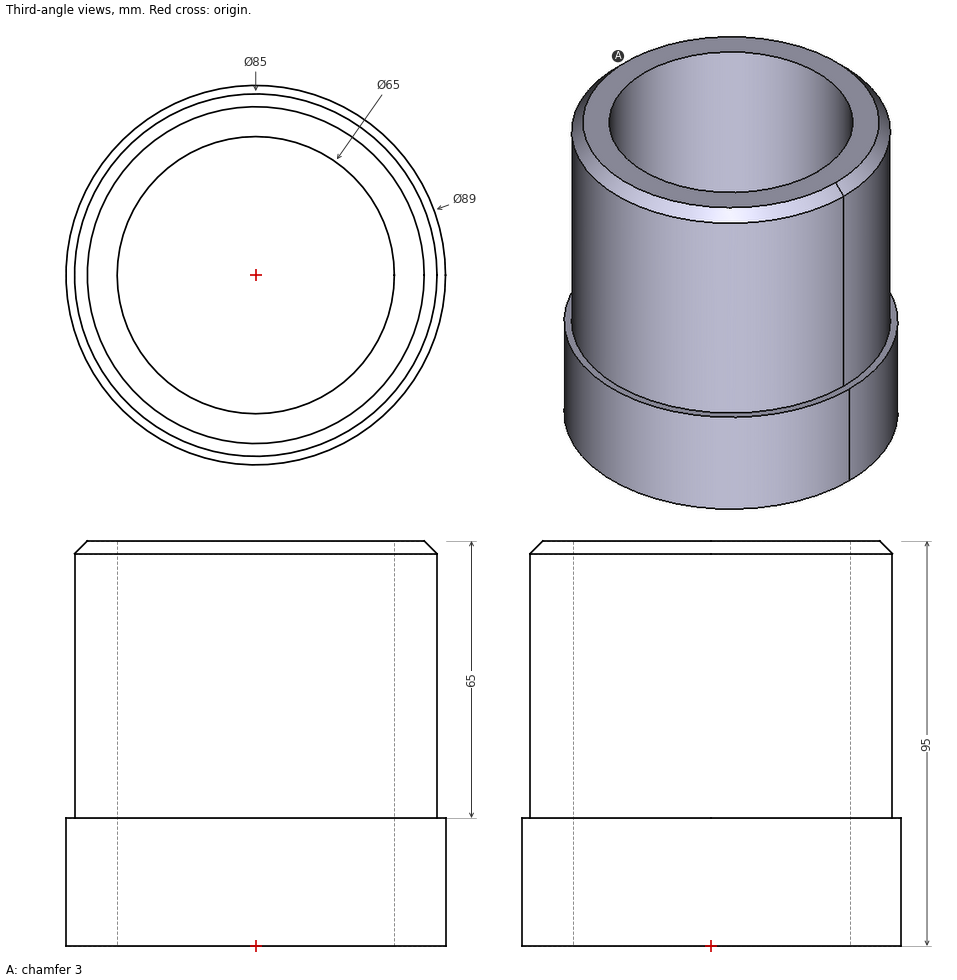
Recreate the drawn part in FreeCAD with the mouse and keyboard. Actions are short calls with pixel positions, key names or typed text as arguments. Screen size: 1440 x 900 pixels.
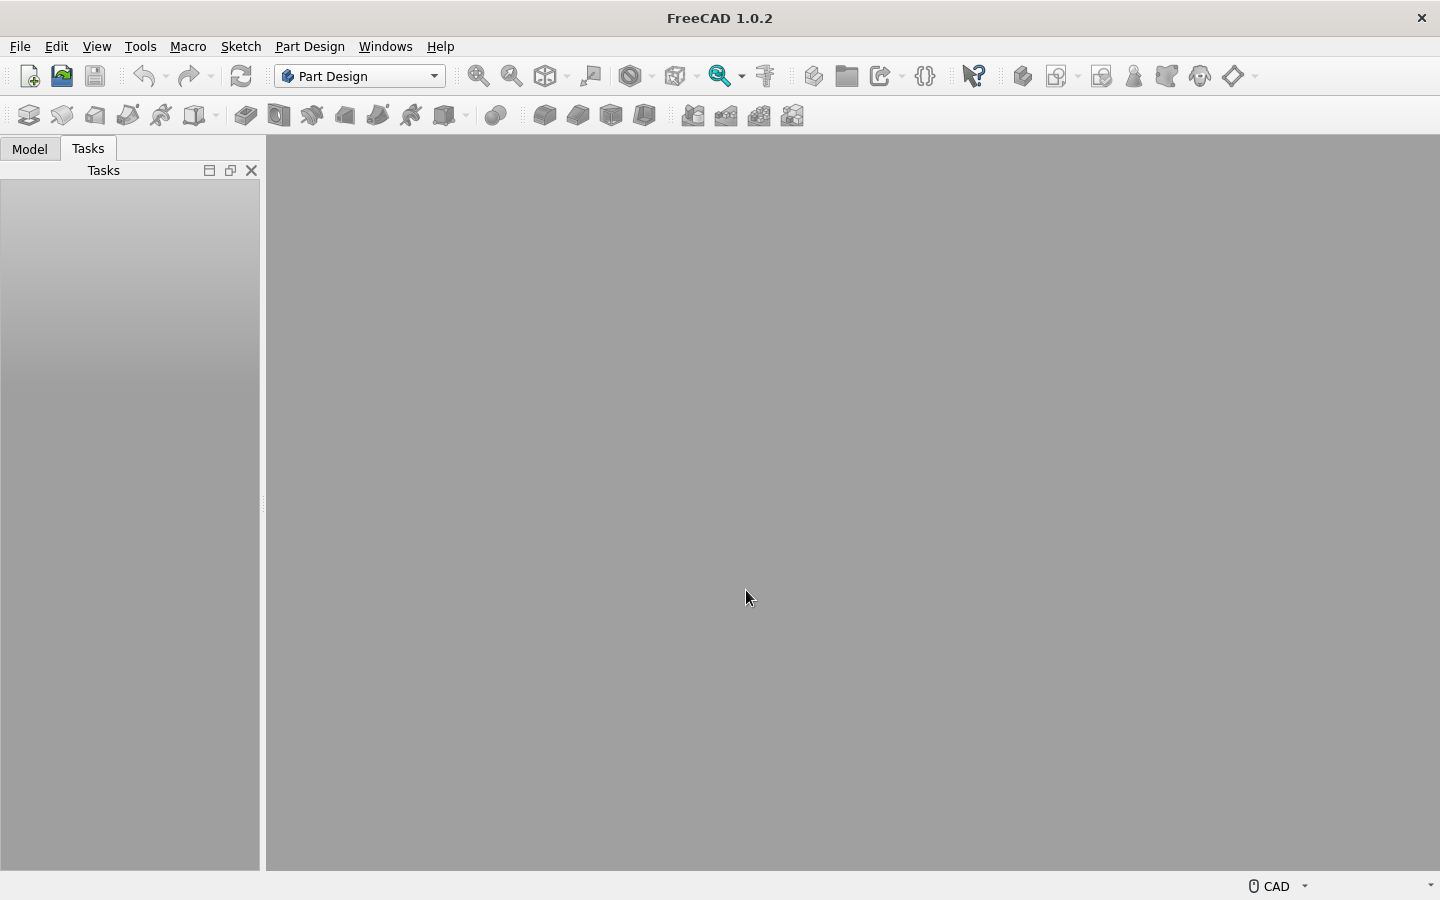
click(29, 76)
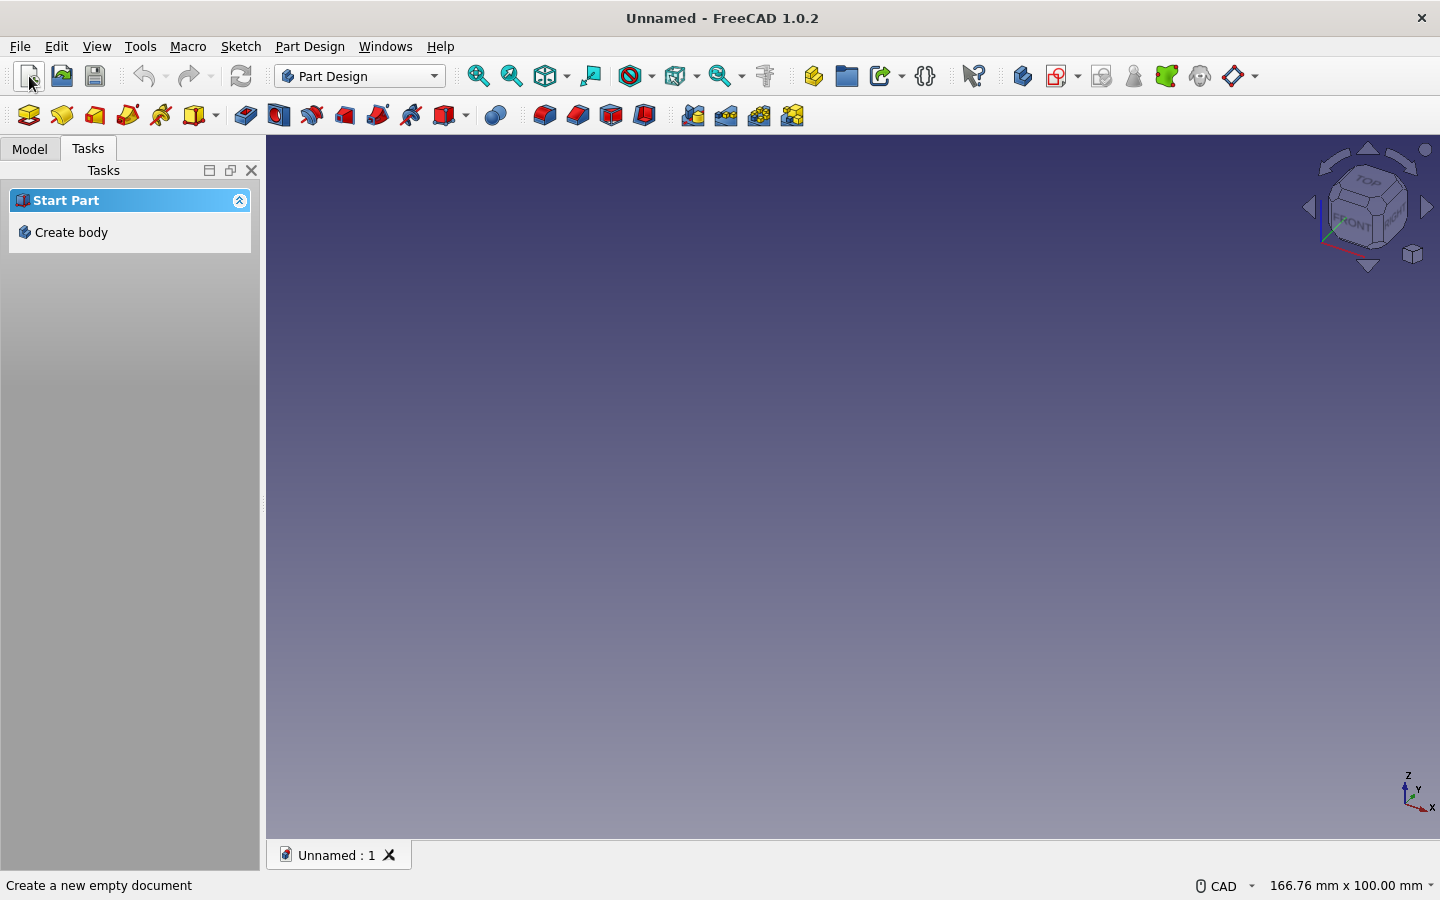
click(1056, 76)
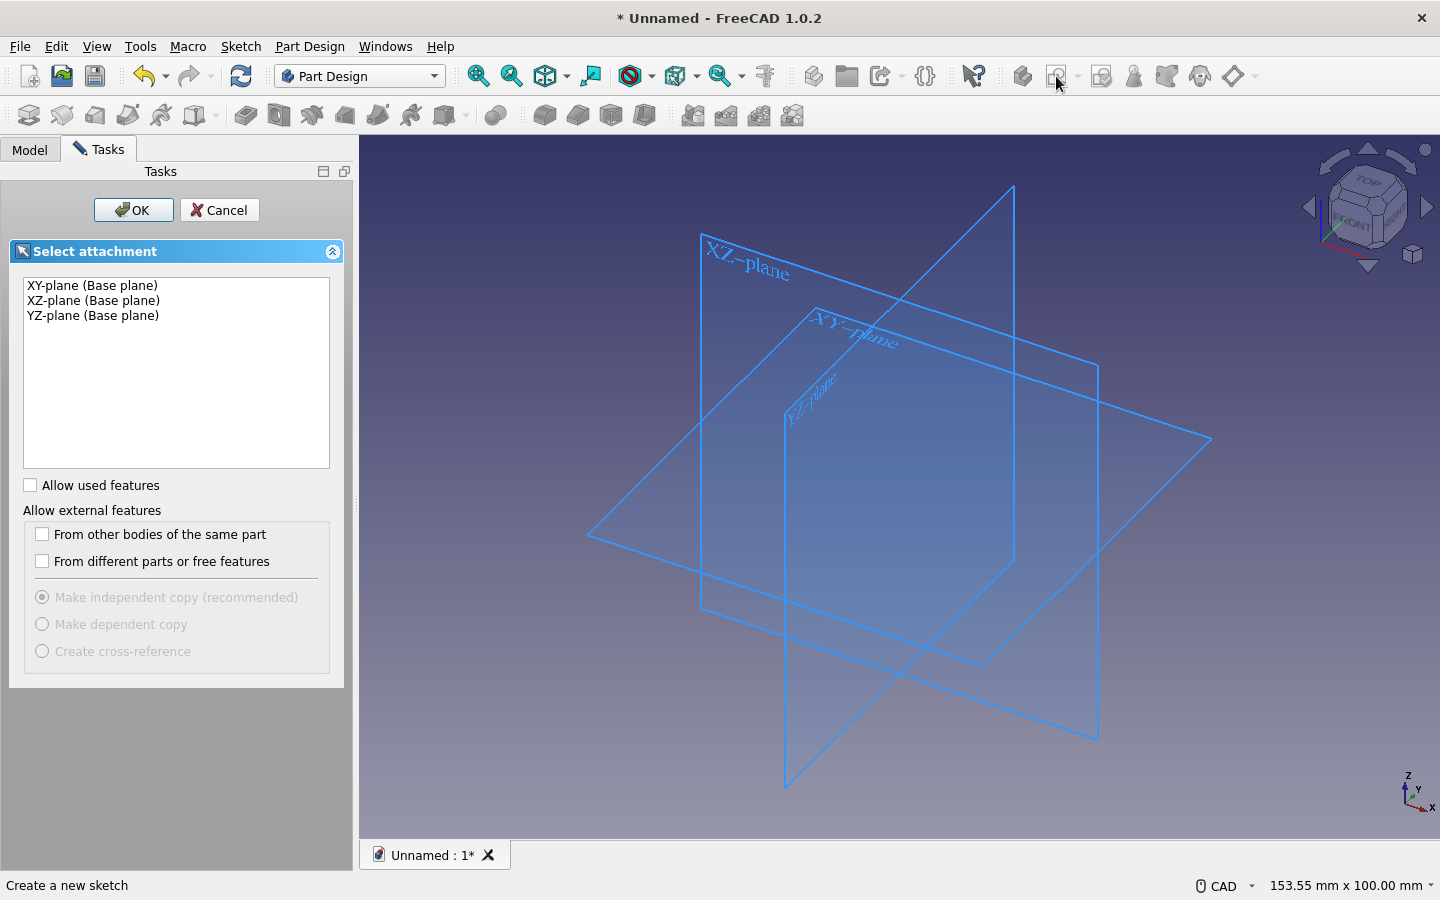
click(84, 286)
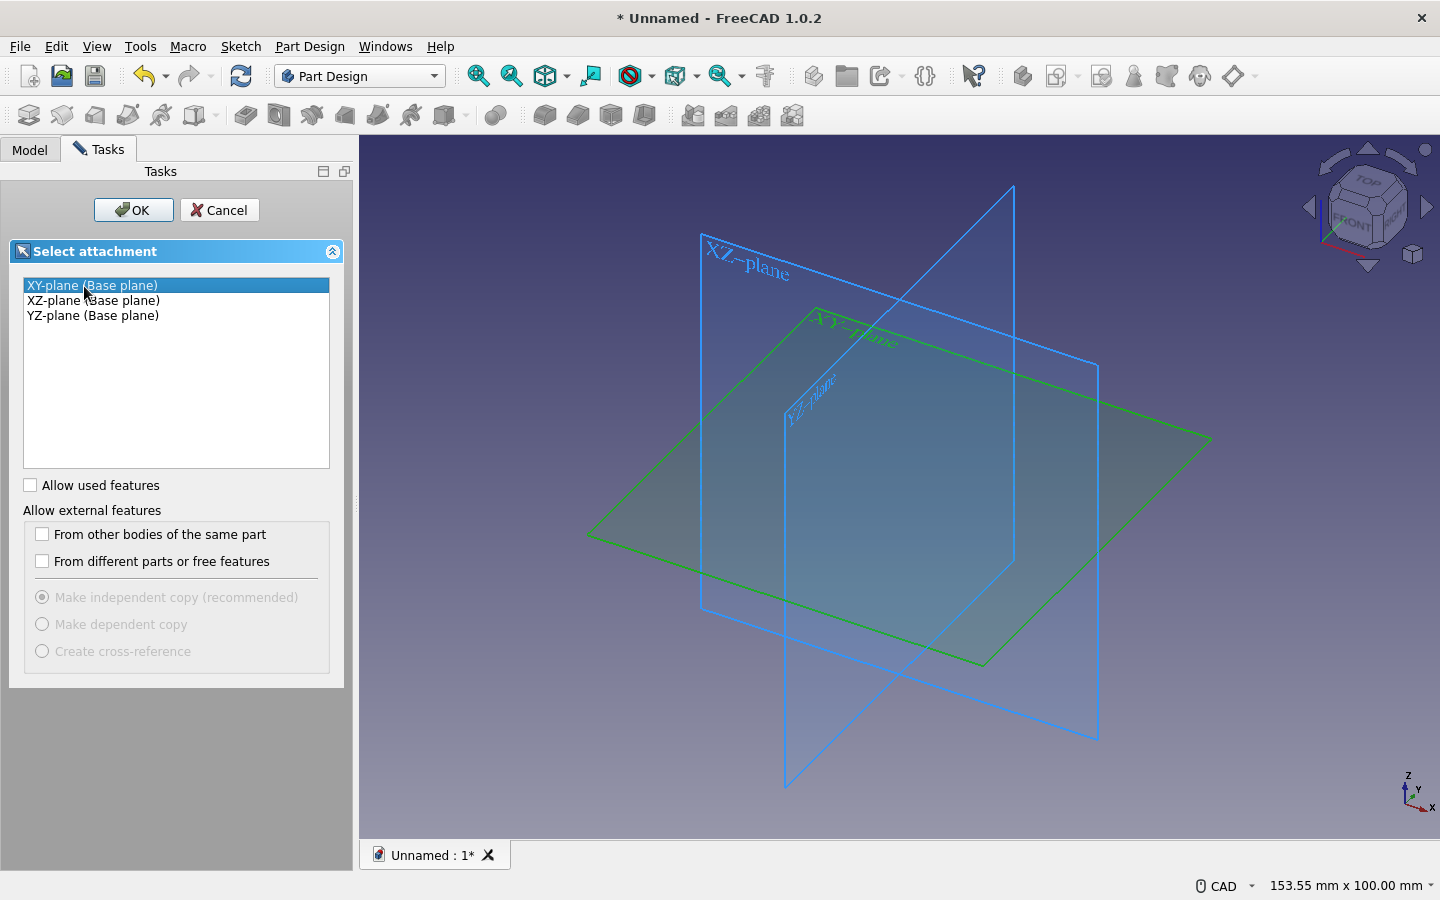
click(134, 210)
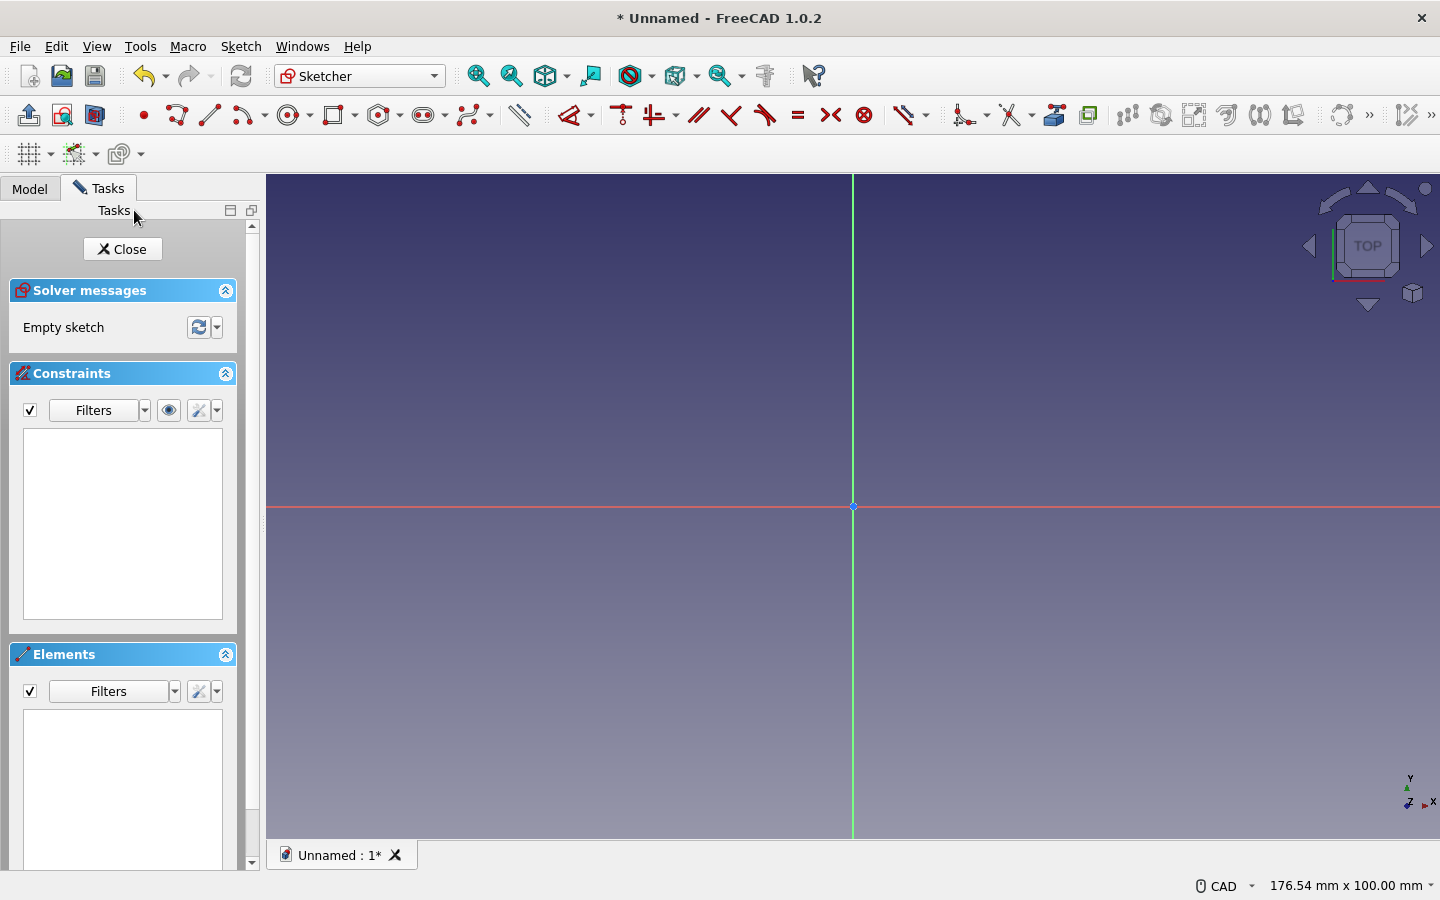
scroll(645, 507, down, 2)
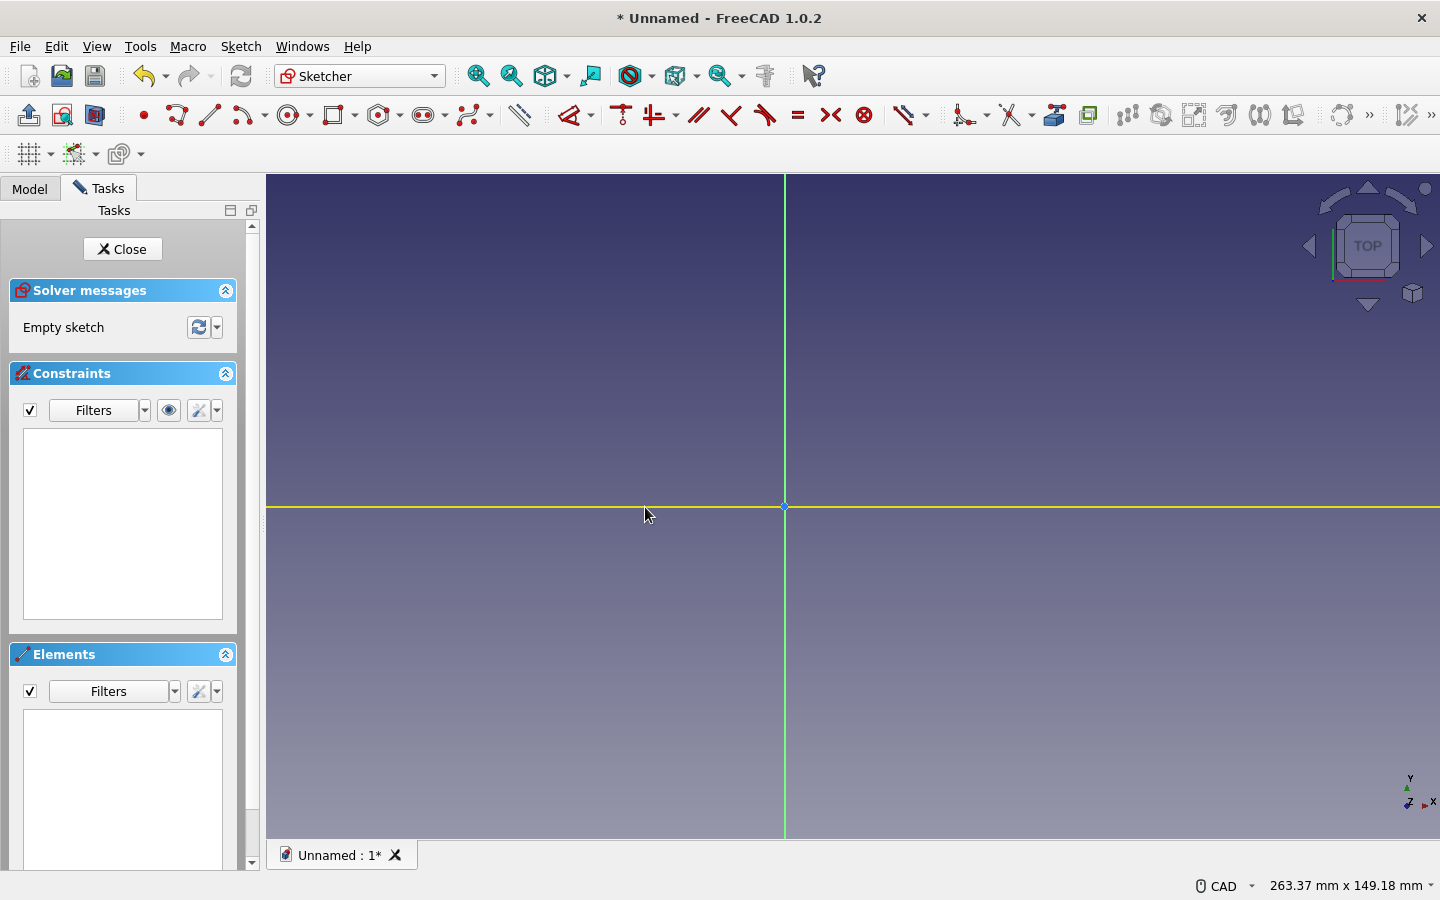
key(g)
key(c)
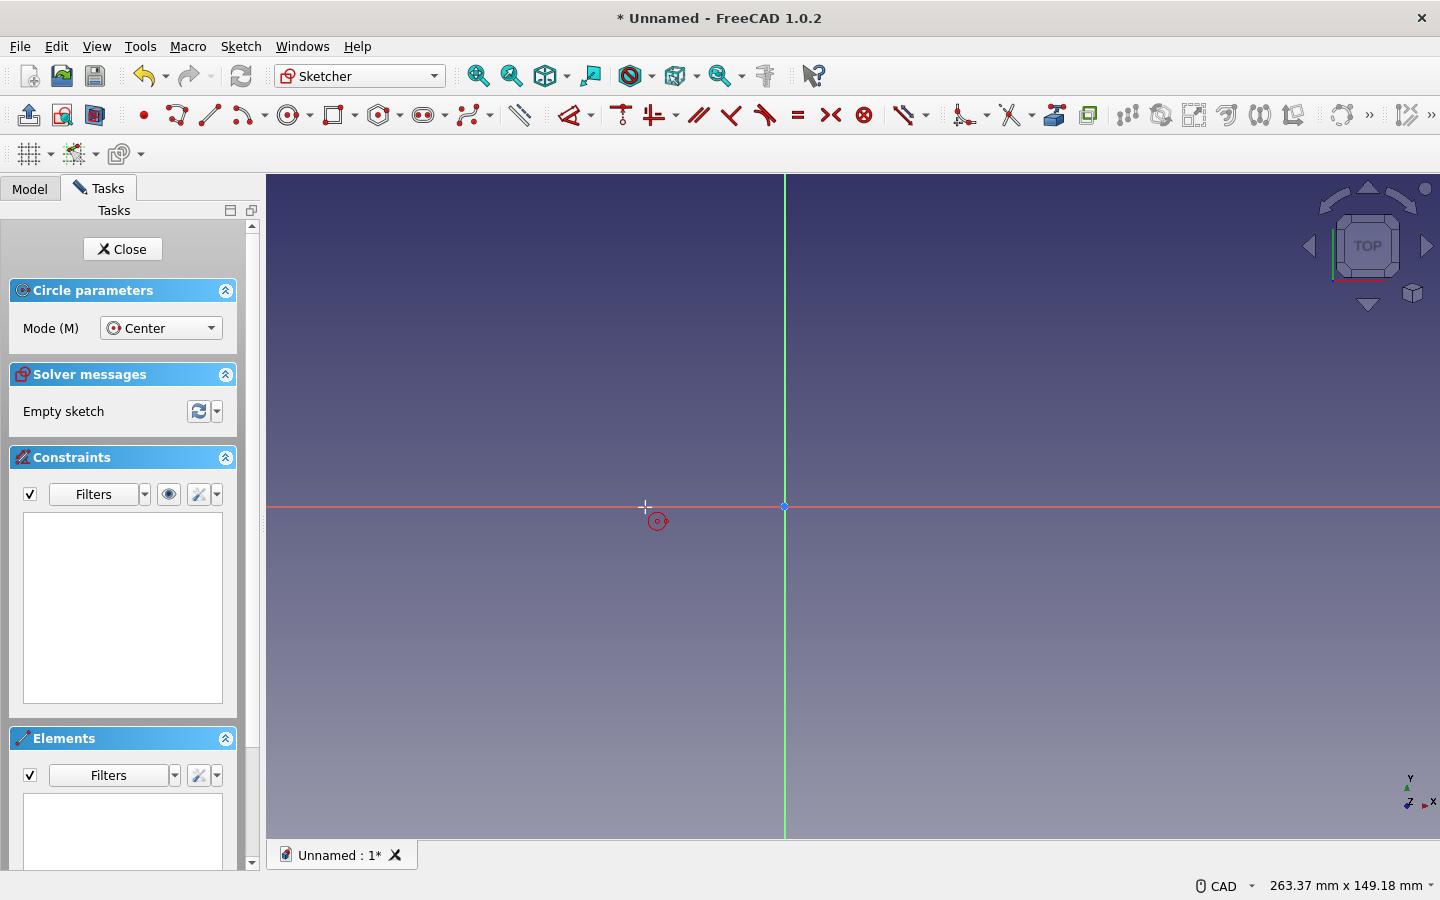
click(785, 507)
click(925, 367)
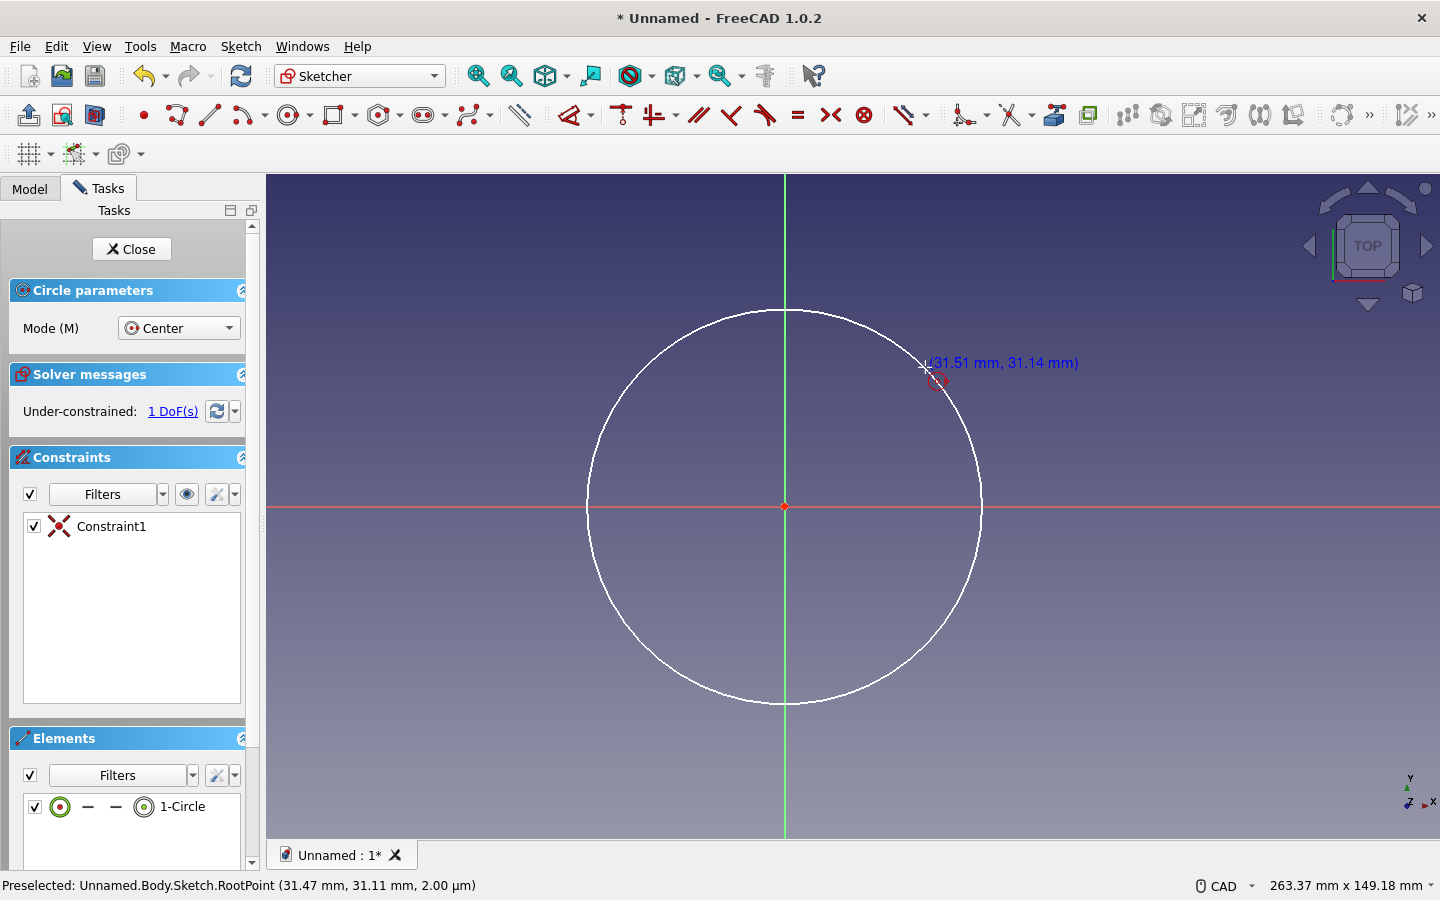
click(785, 507)
click(887, 404)
key(Escape)